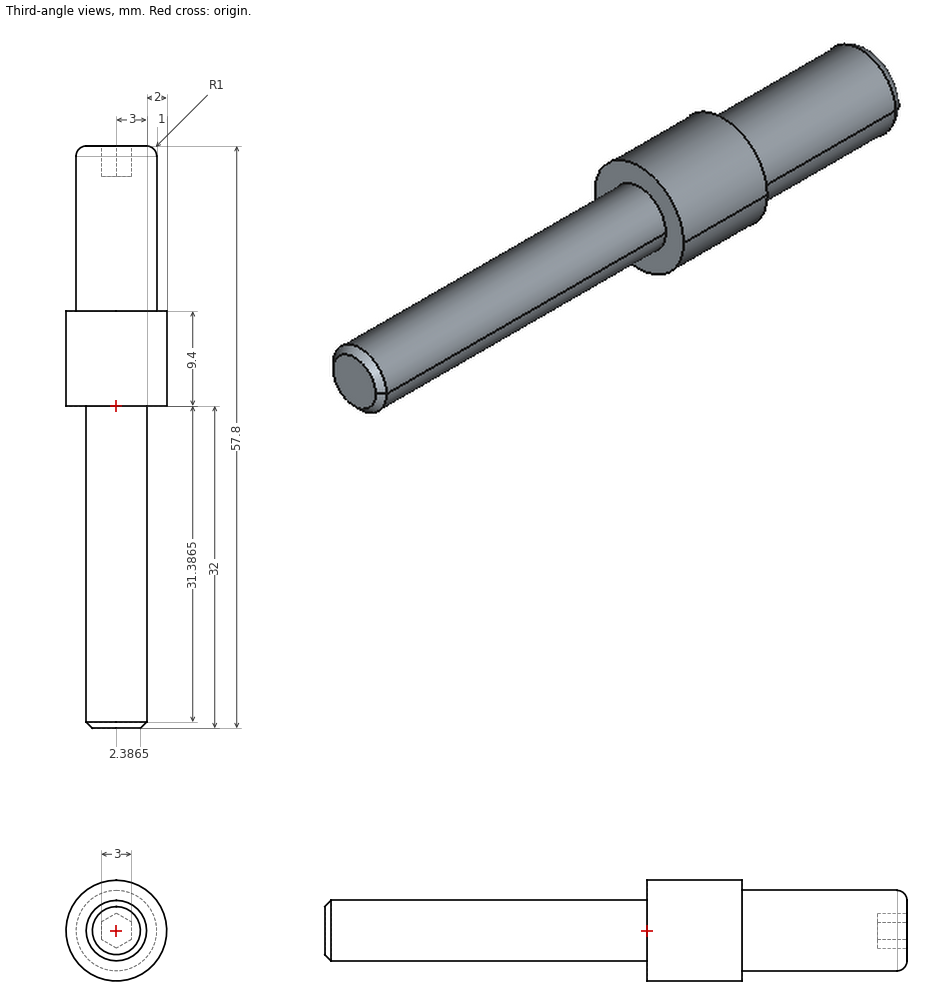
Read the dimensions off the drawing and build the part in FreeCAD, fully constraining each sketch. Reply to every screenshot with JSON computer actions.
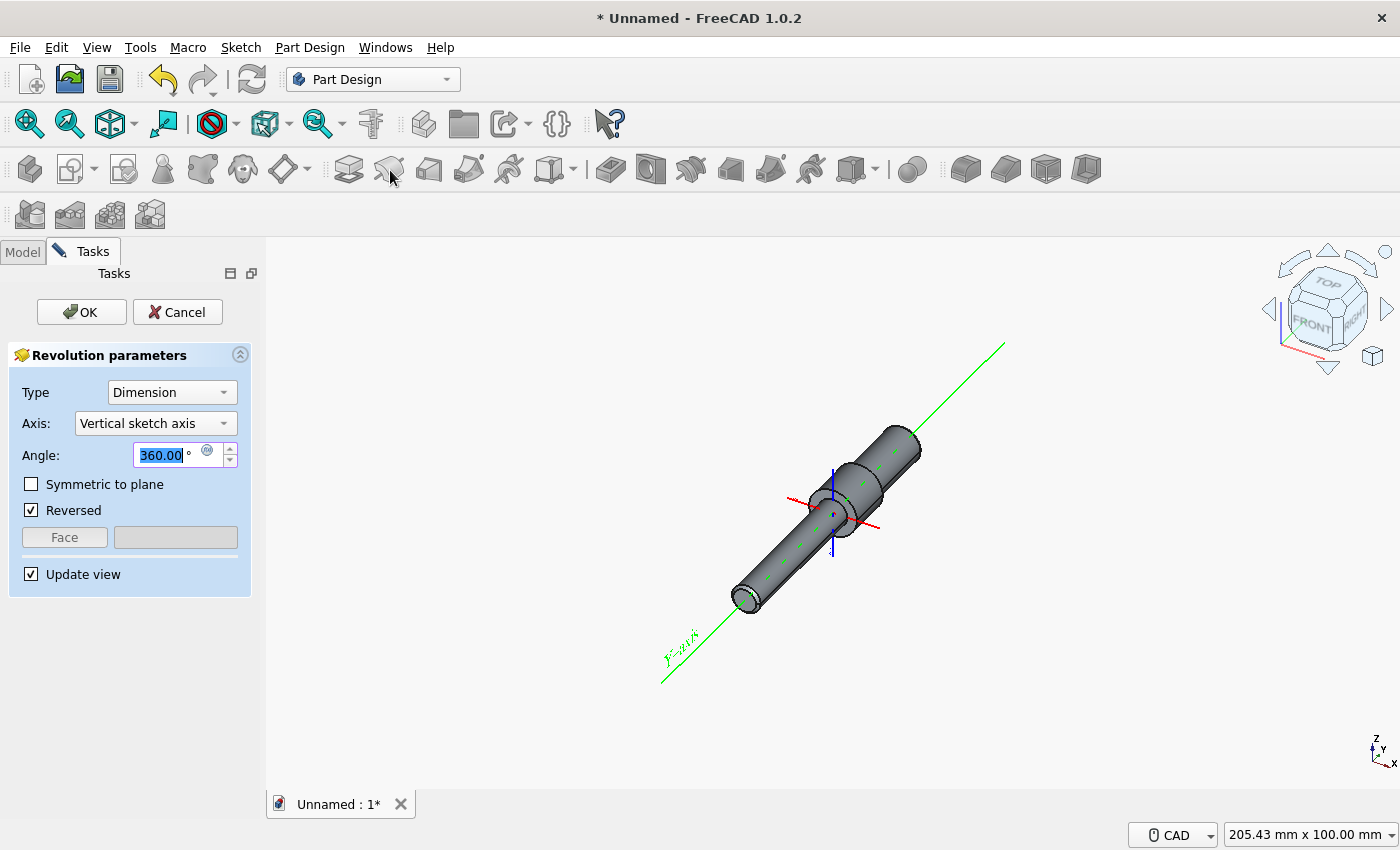
{"action": "left_click", "coordinate": [82, 312]}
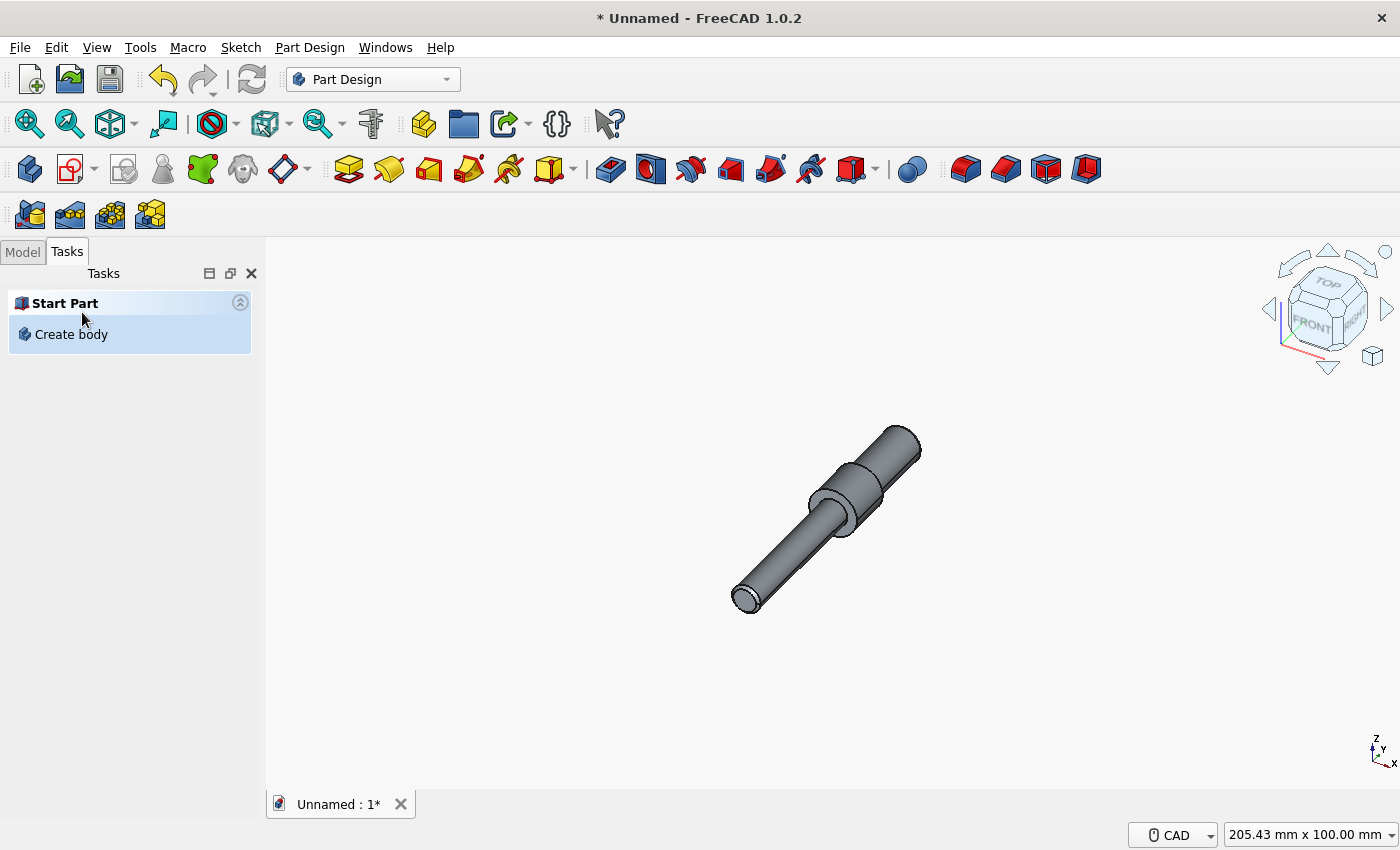
{"action": "left_click", "coordinate": [30, 124]}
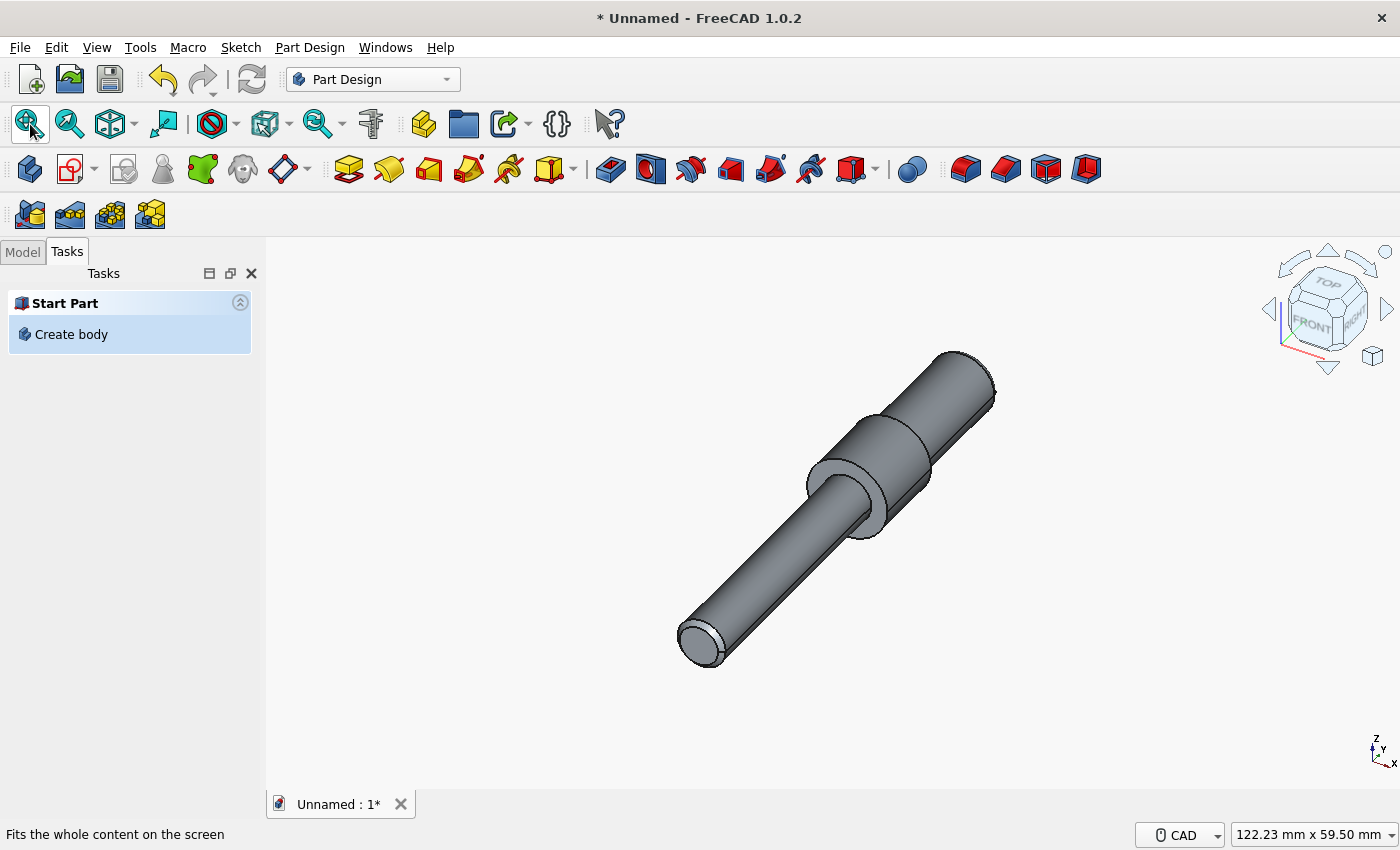
{"action": "key", "text": "4"}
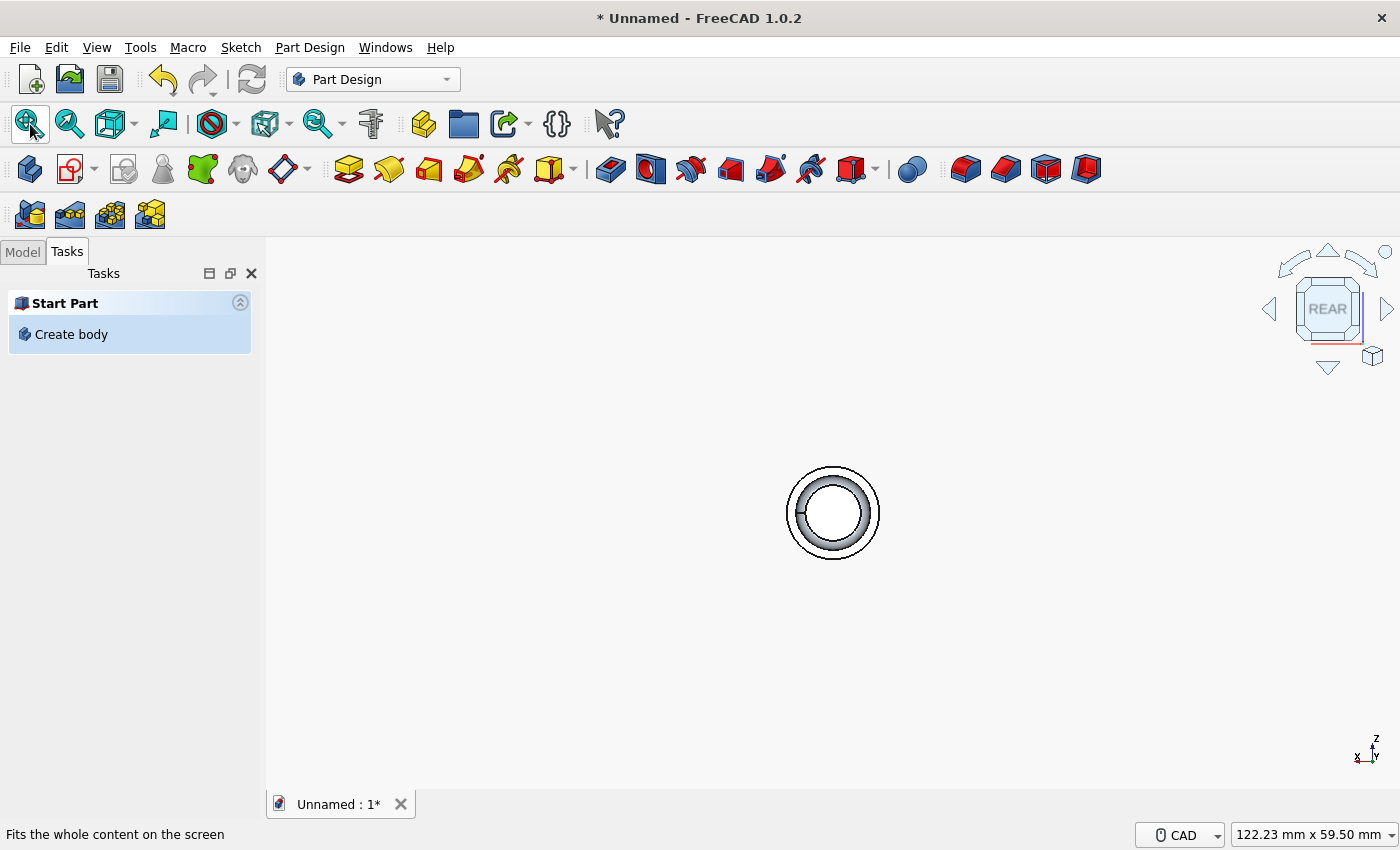
{"action": "left_click", "coordinate": [30, 124]}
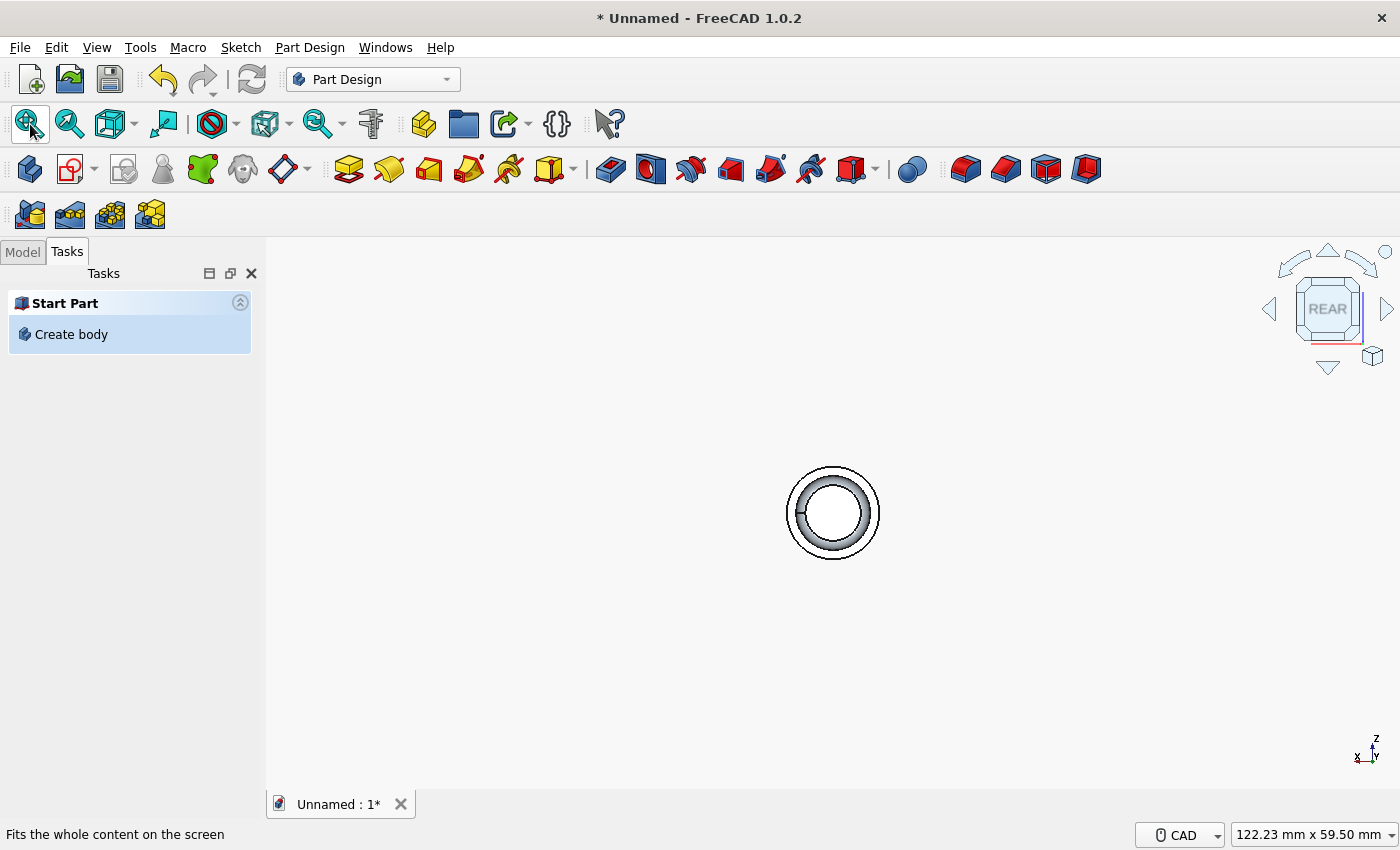
{"action": "left_click", "coordinate": [833, 512]}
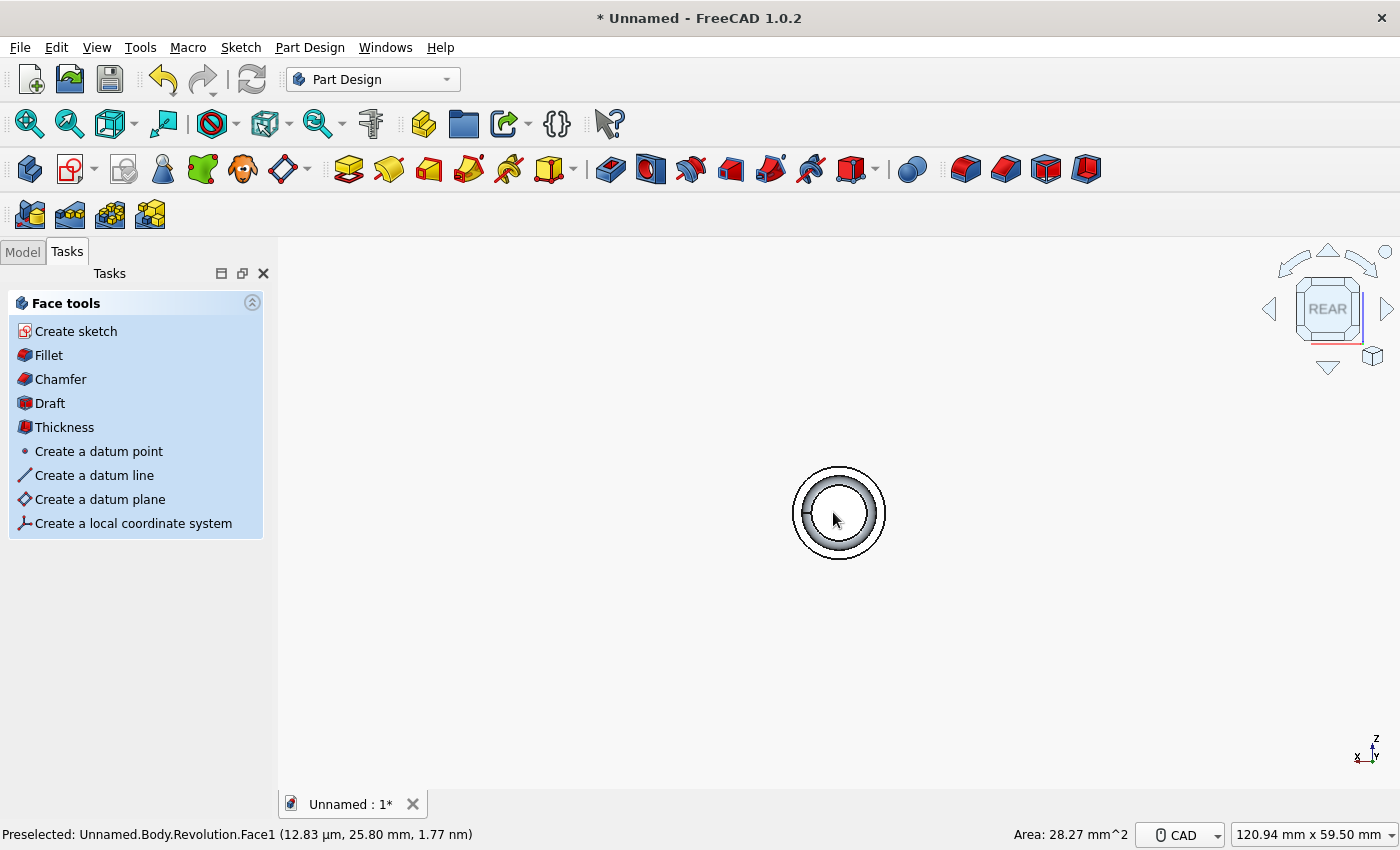
{"action": "left_click", "coordinate": [70, 170]}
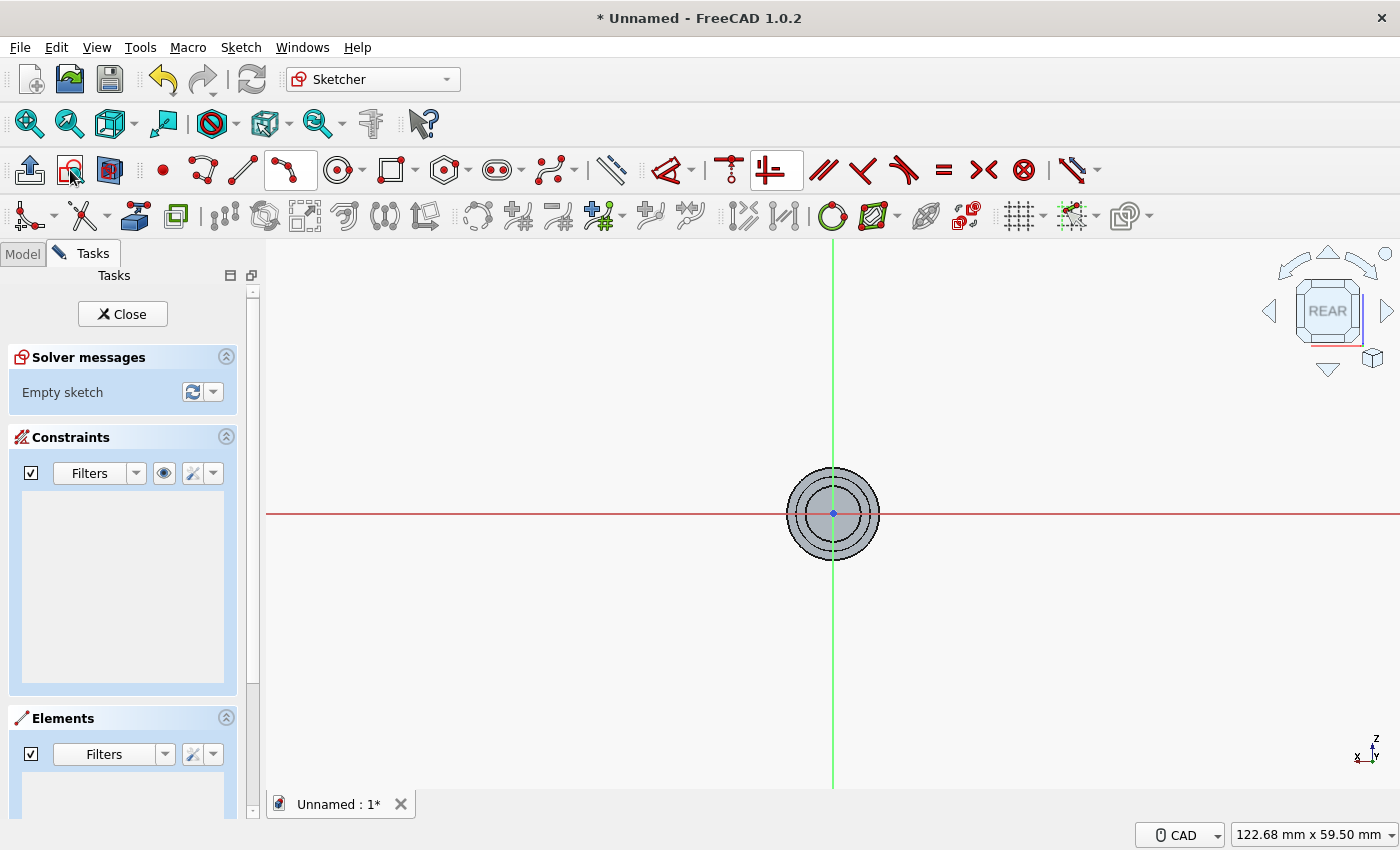
{"action": "scroll", "coordinate": [840, 514], "scroll_direction": "up", "scroll_amount": 12}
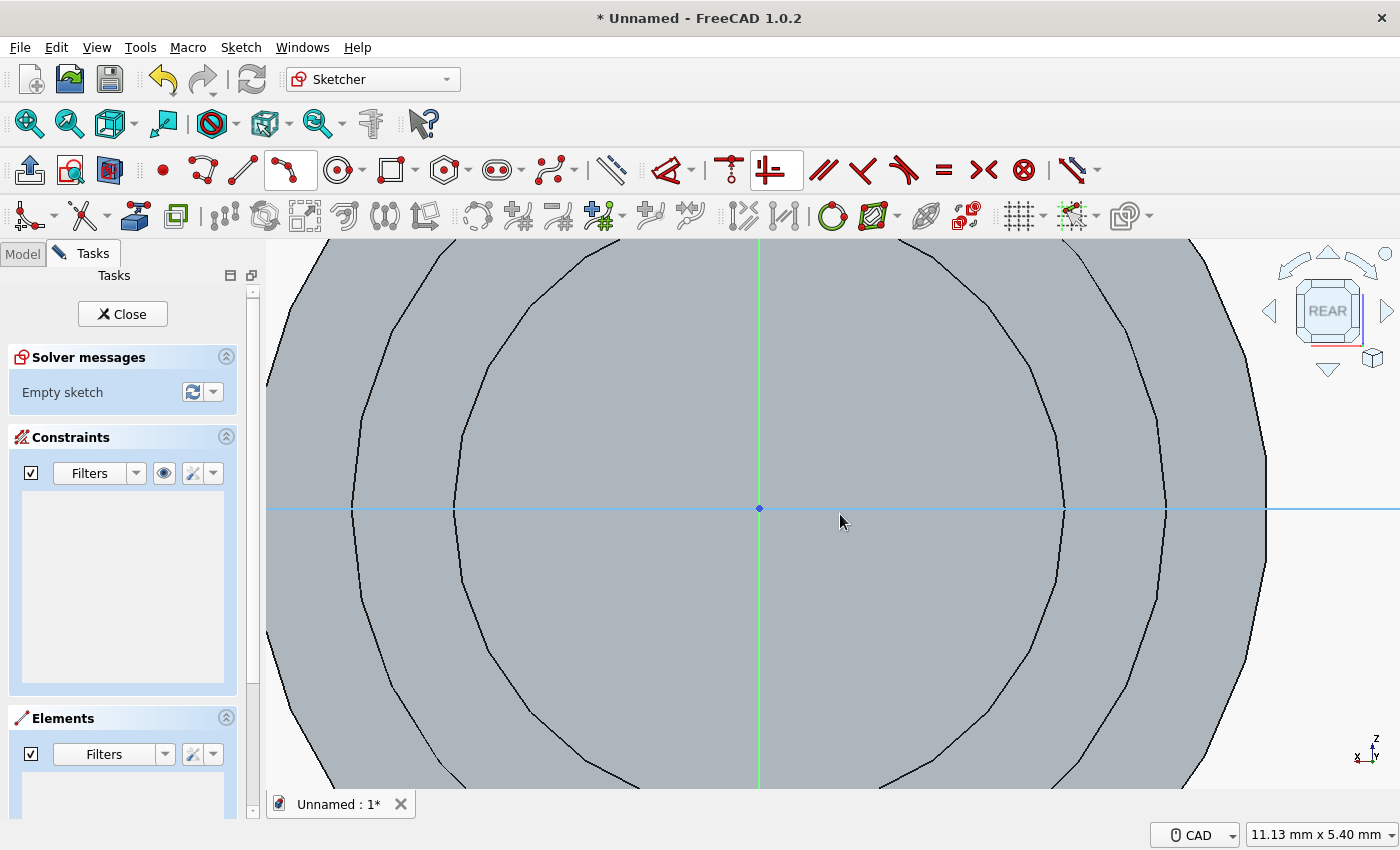
{"action": "left_click", "coordinate": [444, 170]}